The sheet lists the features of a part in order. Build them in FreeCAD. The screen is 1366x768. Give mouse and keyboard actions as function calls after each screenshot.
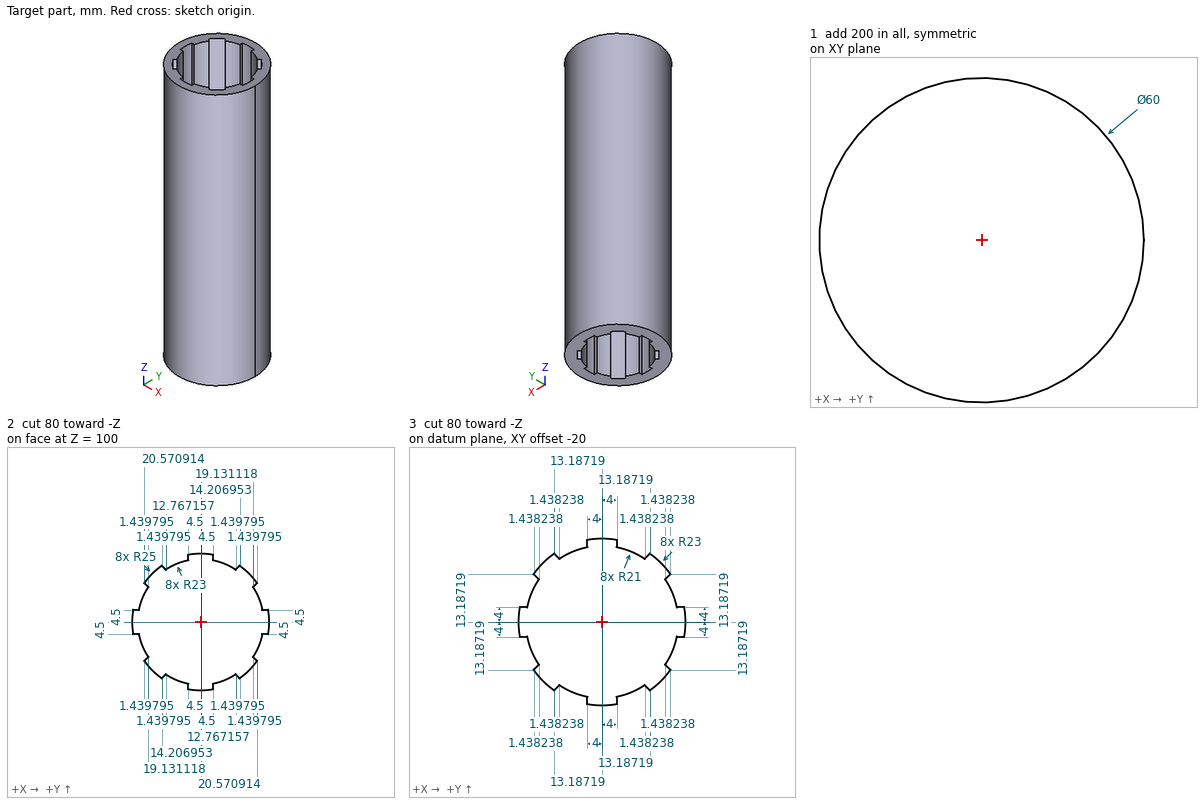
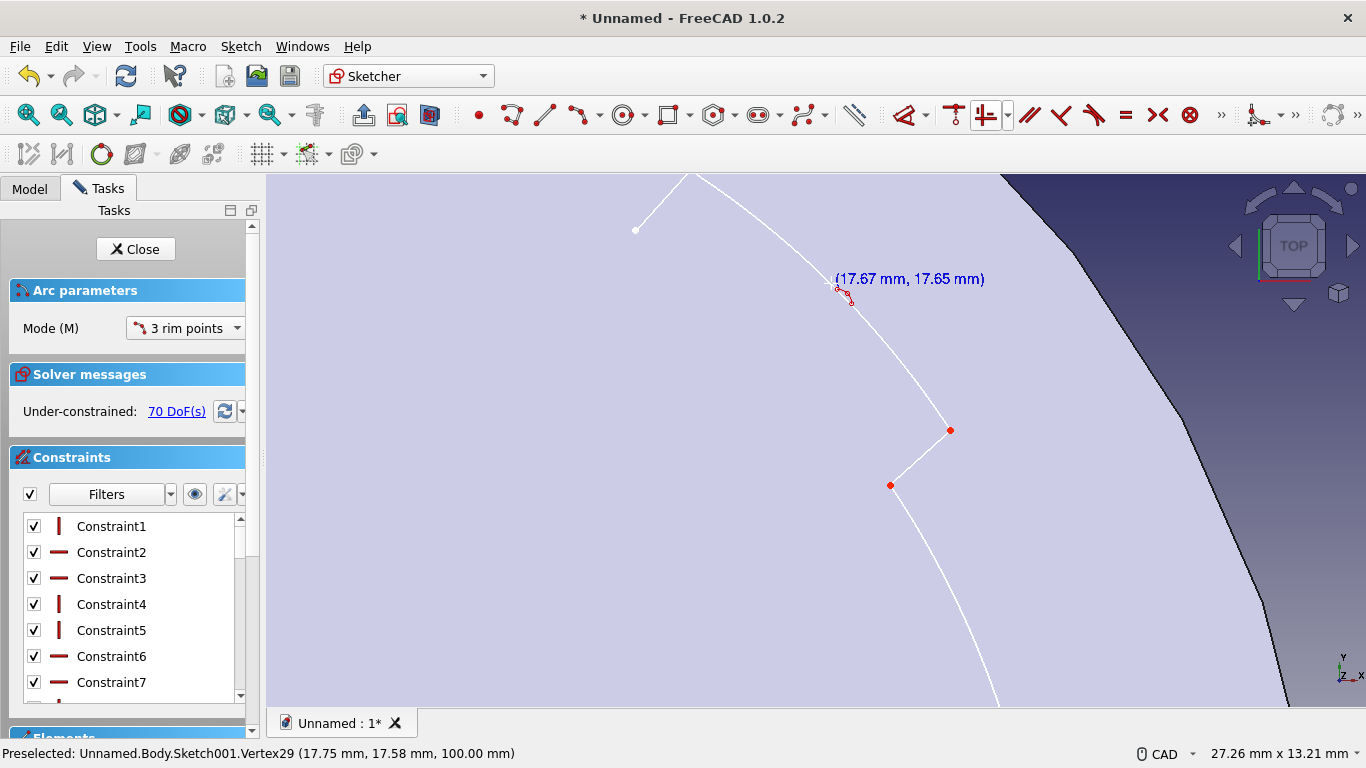
click(636, 231)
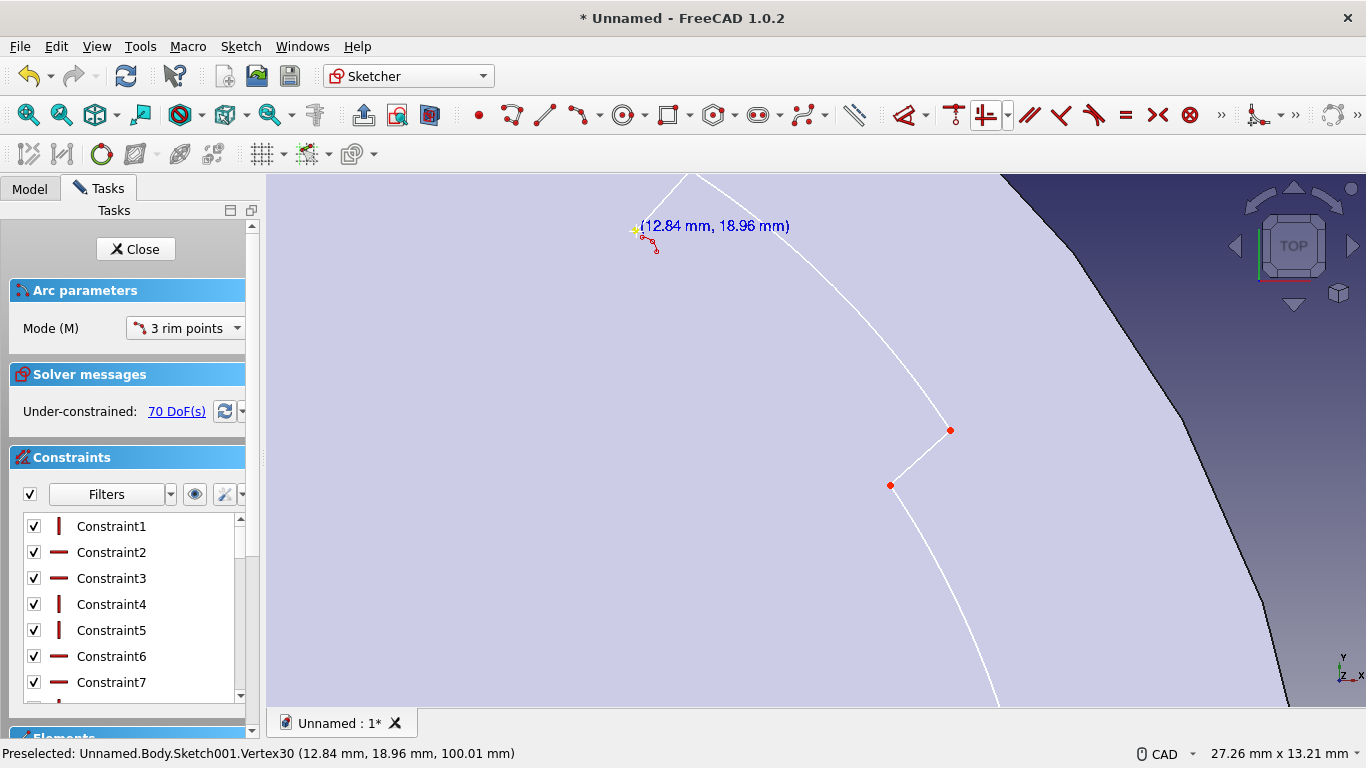
scroll(872, 330, down, 9)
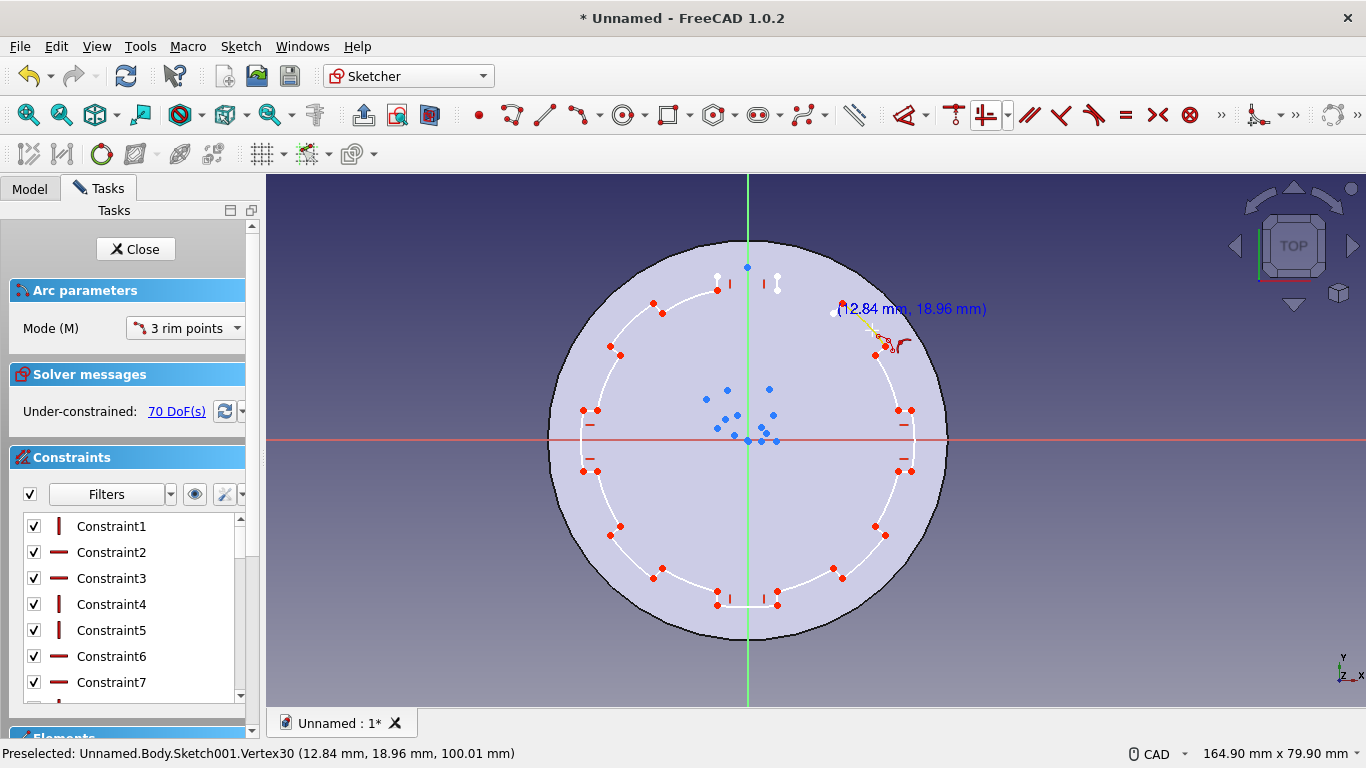
scroll(778, 290, up, 5)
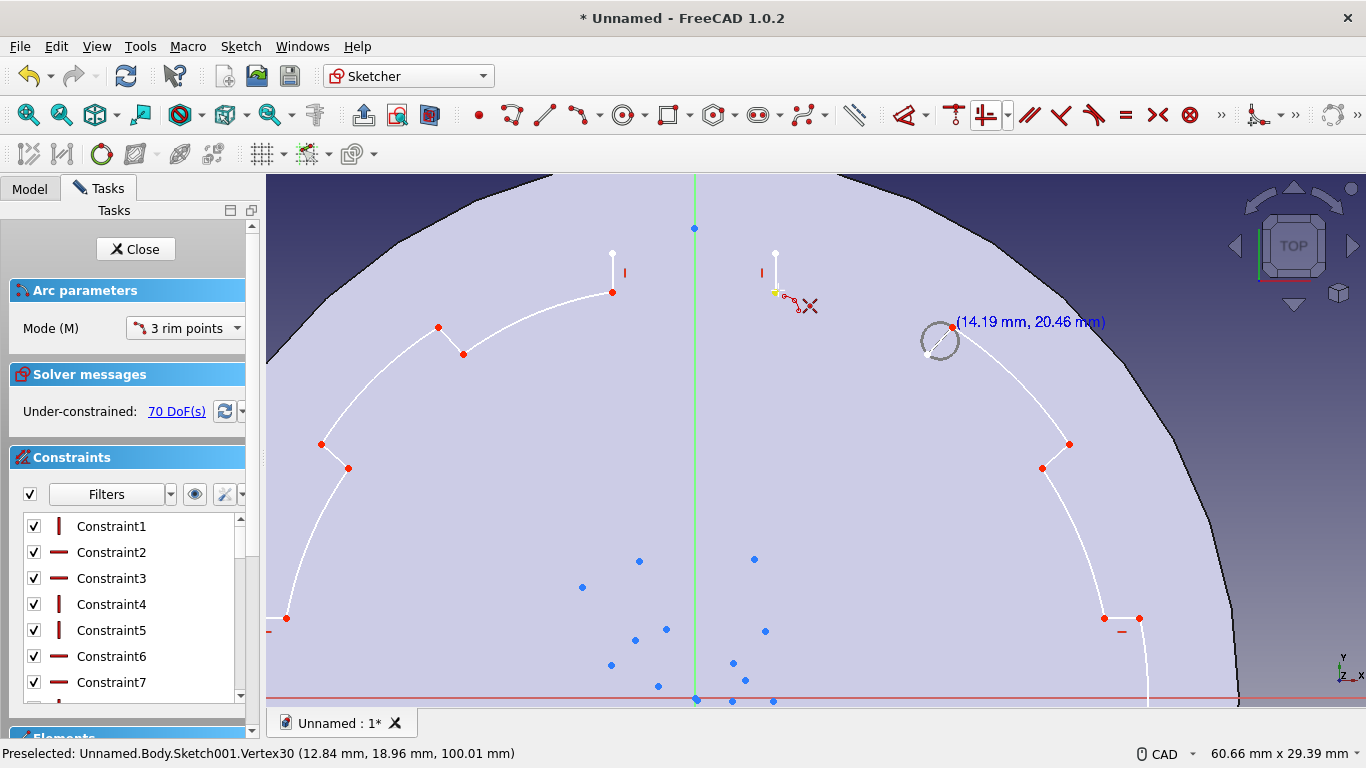
click(776, 292)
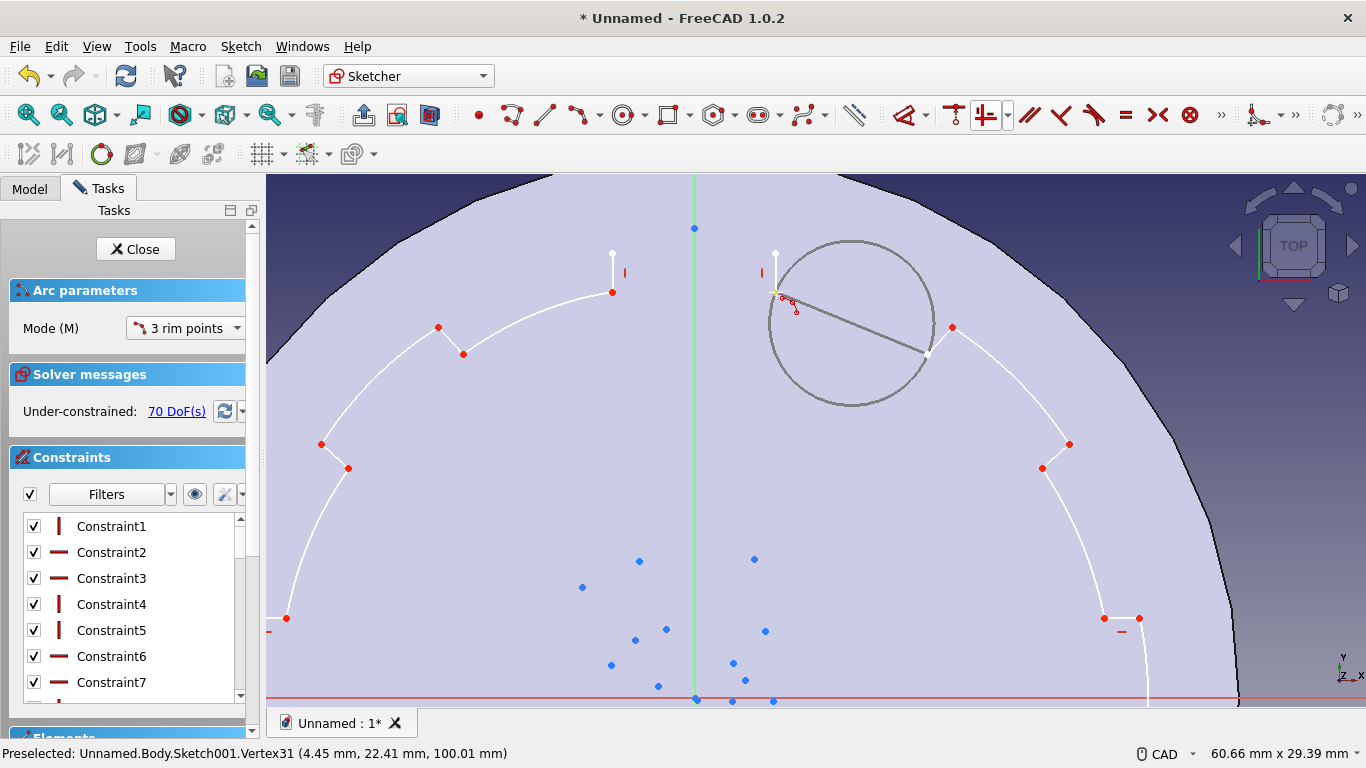
scroll(855, 313, up, 4)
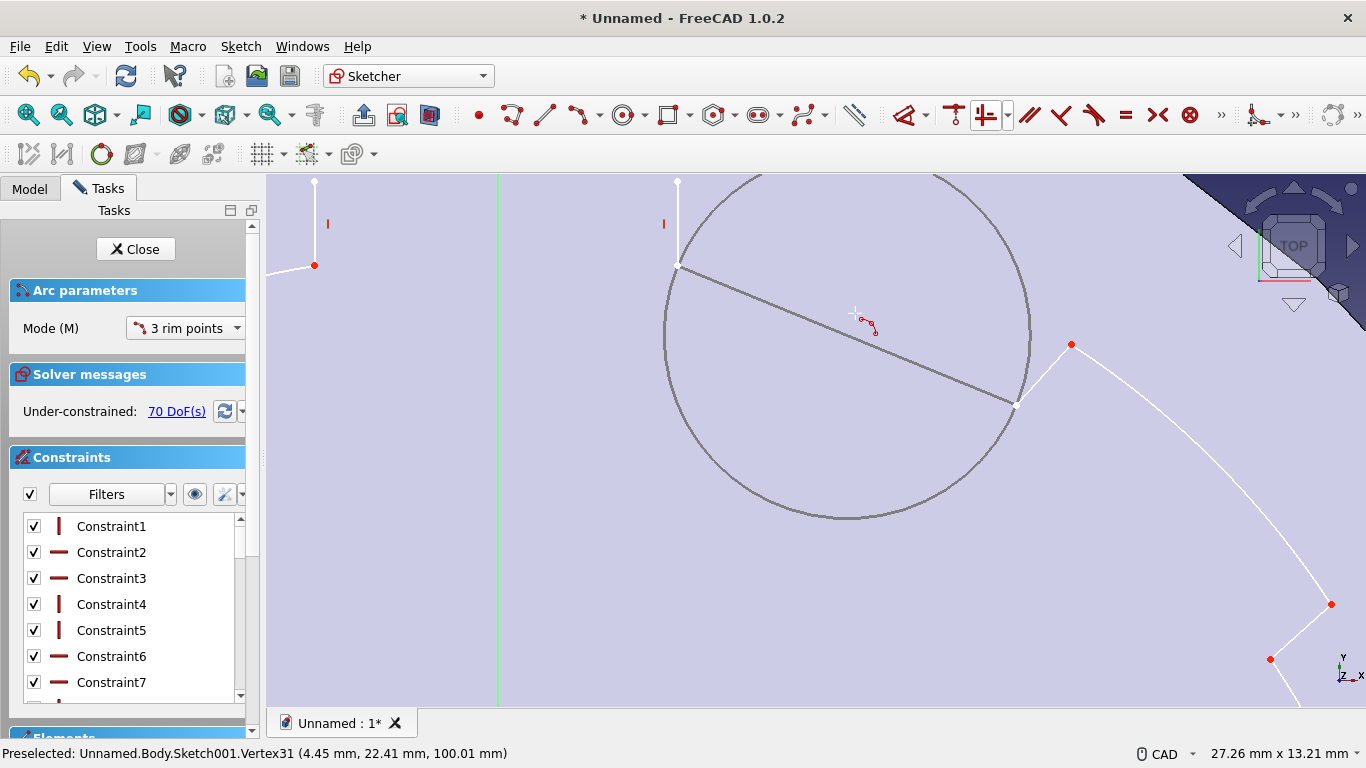
click(854, 313)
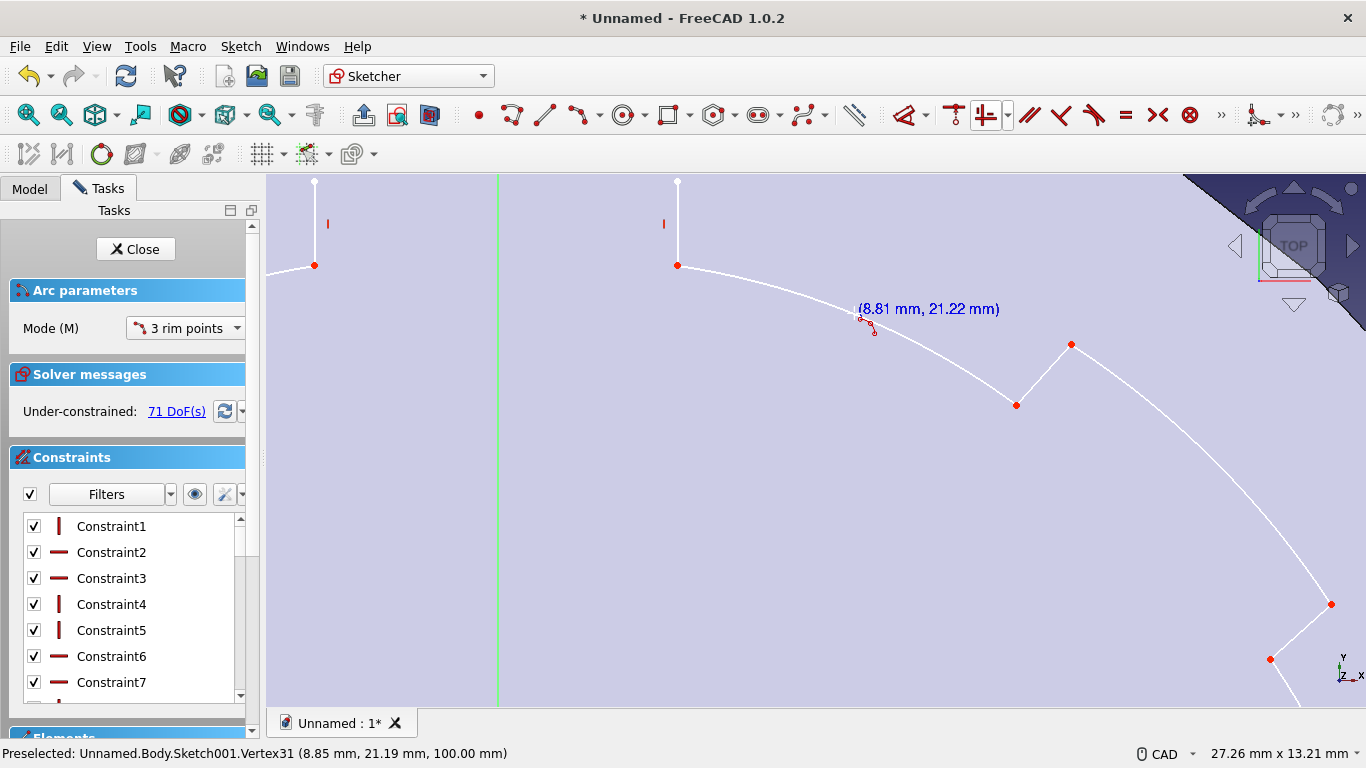
scroll(797, 296, down, 9)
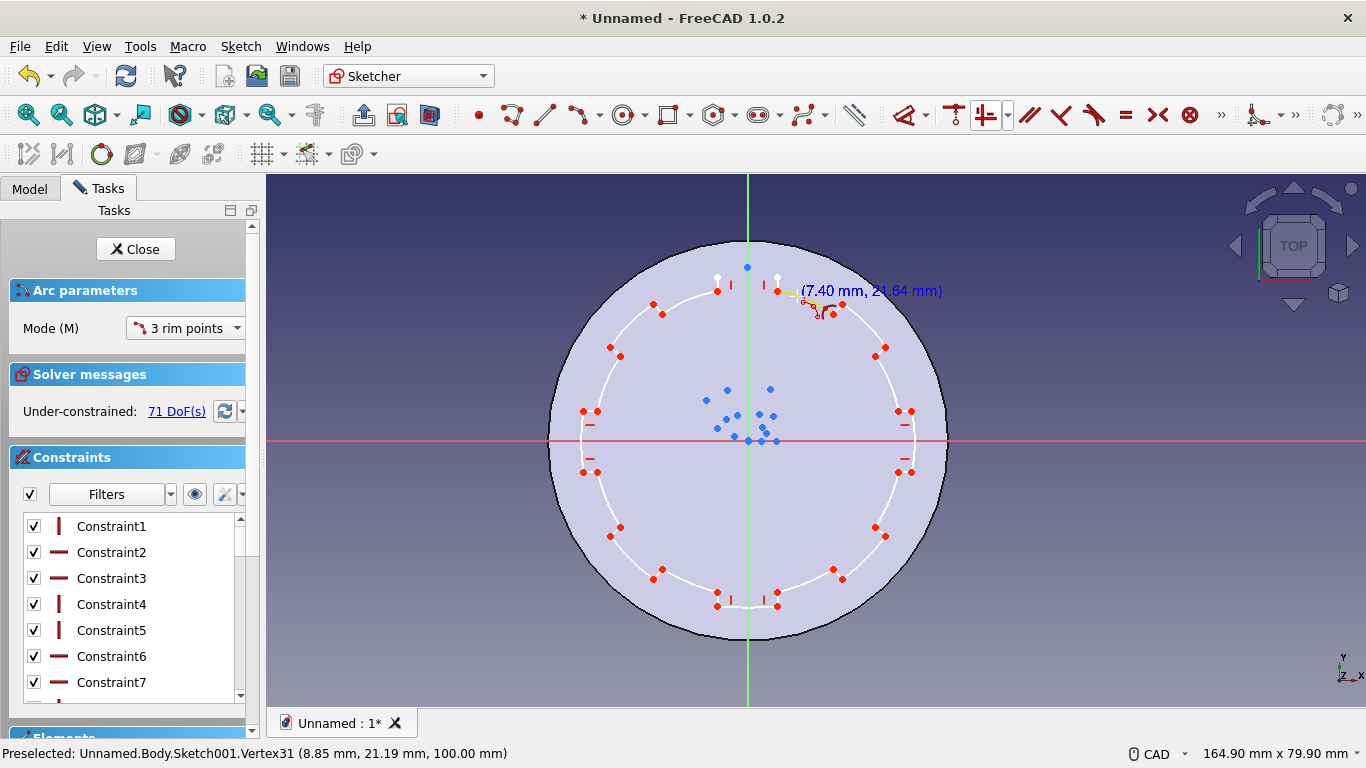
scroll(778, 277, up, 5)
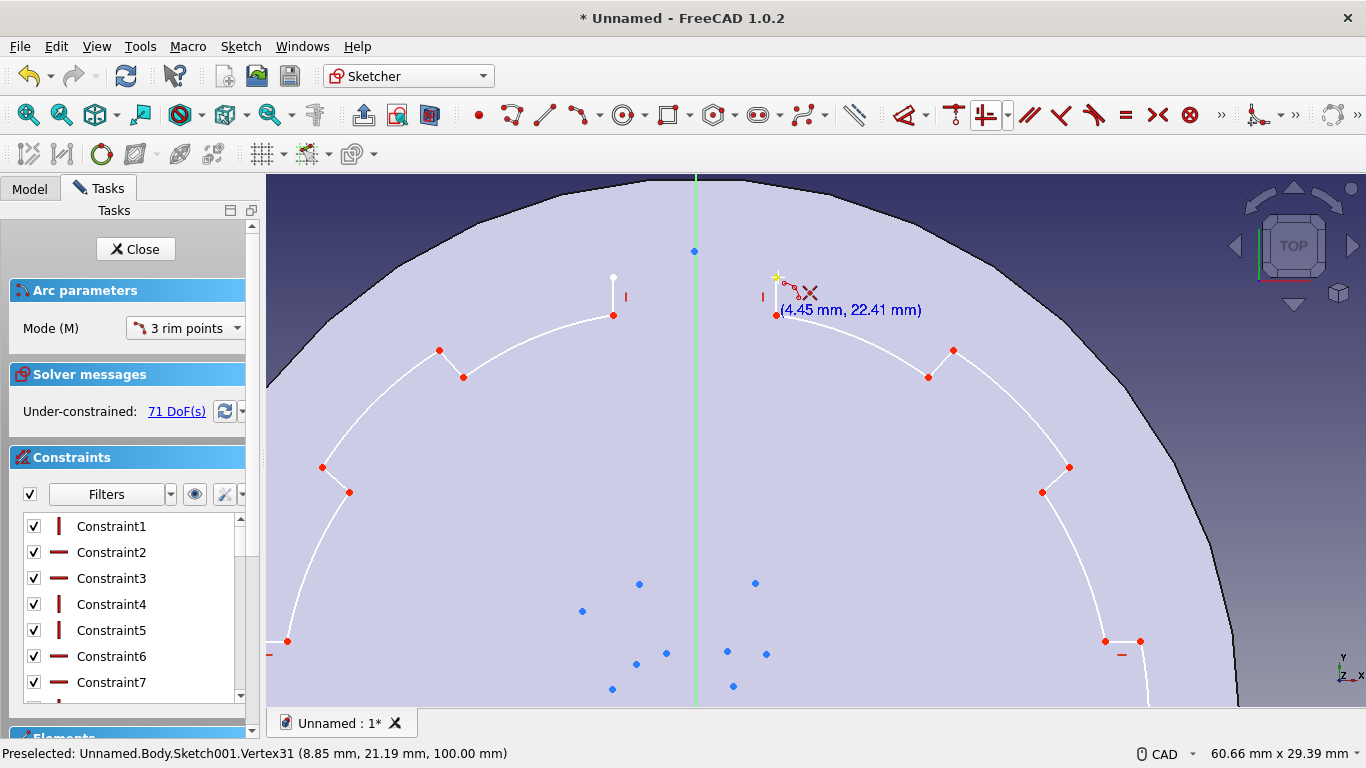
click(776, 277)
click(613, 277)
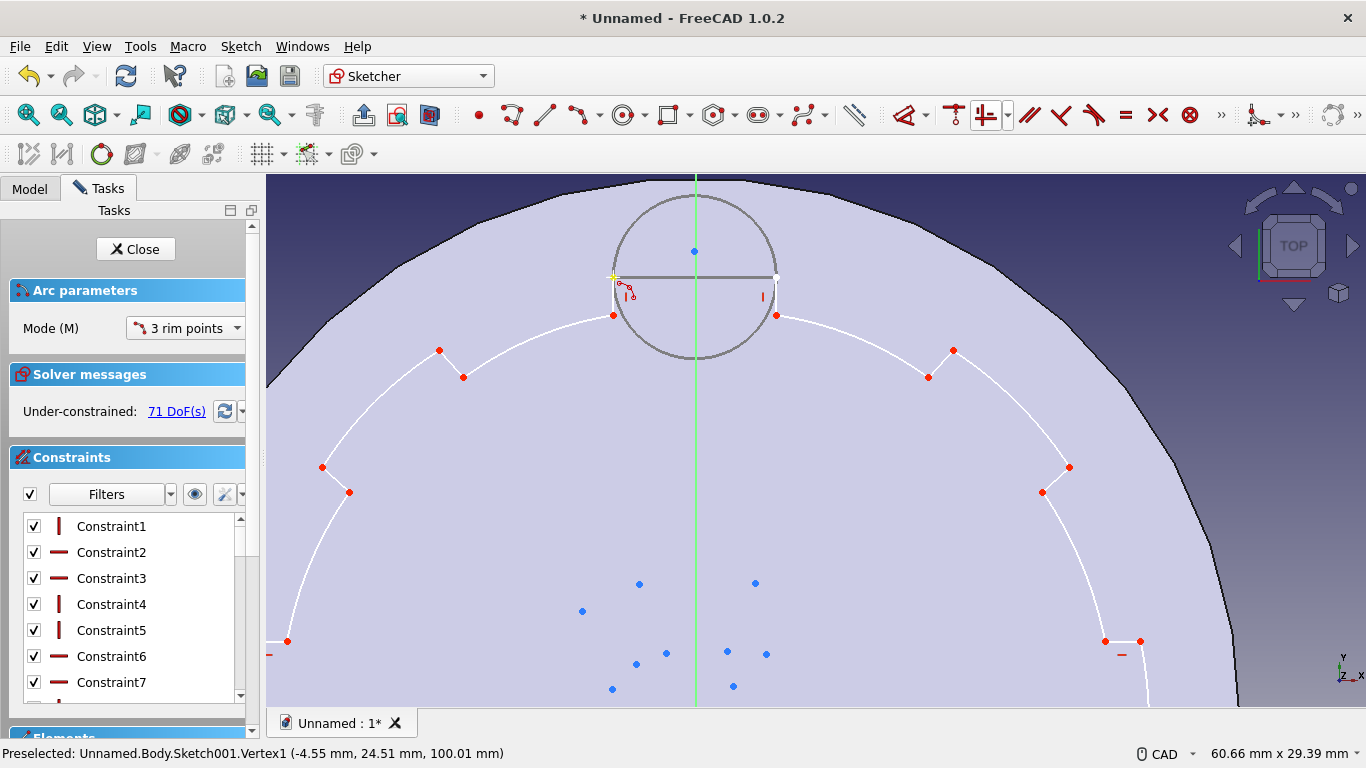
scroll(712, 269, up, 5)